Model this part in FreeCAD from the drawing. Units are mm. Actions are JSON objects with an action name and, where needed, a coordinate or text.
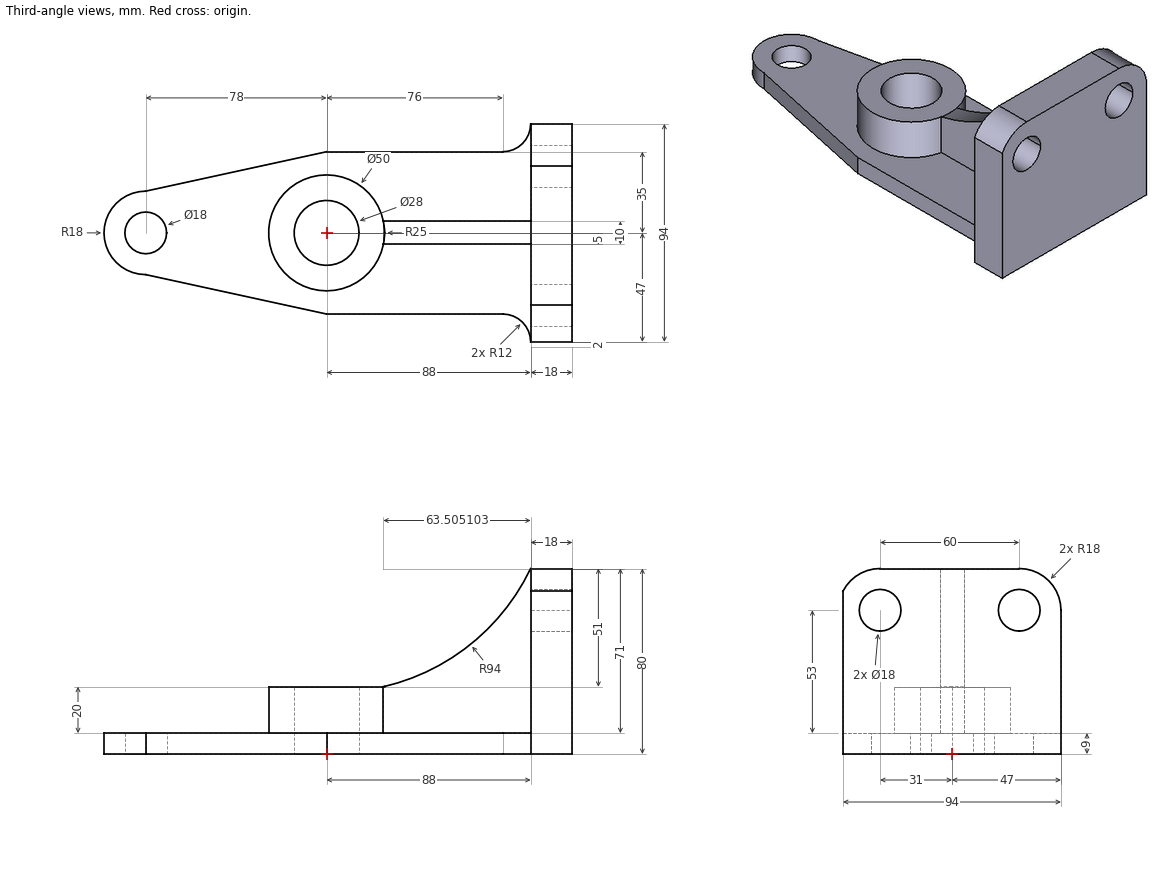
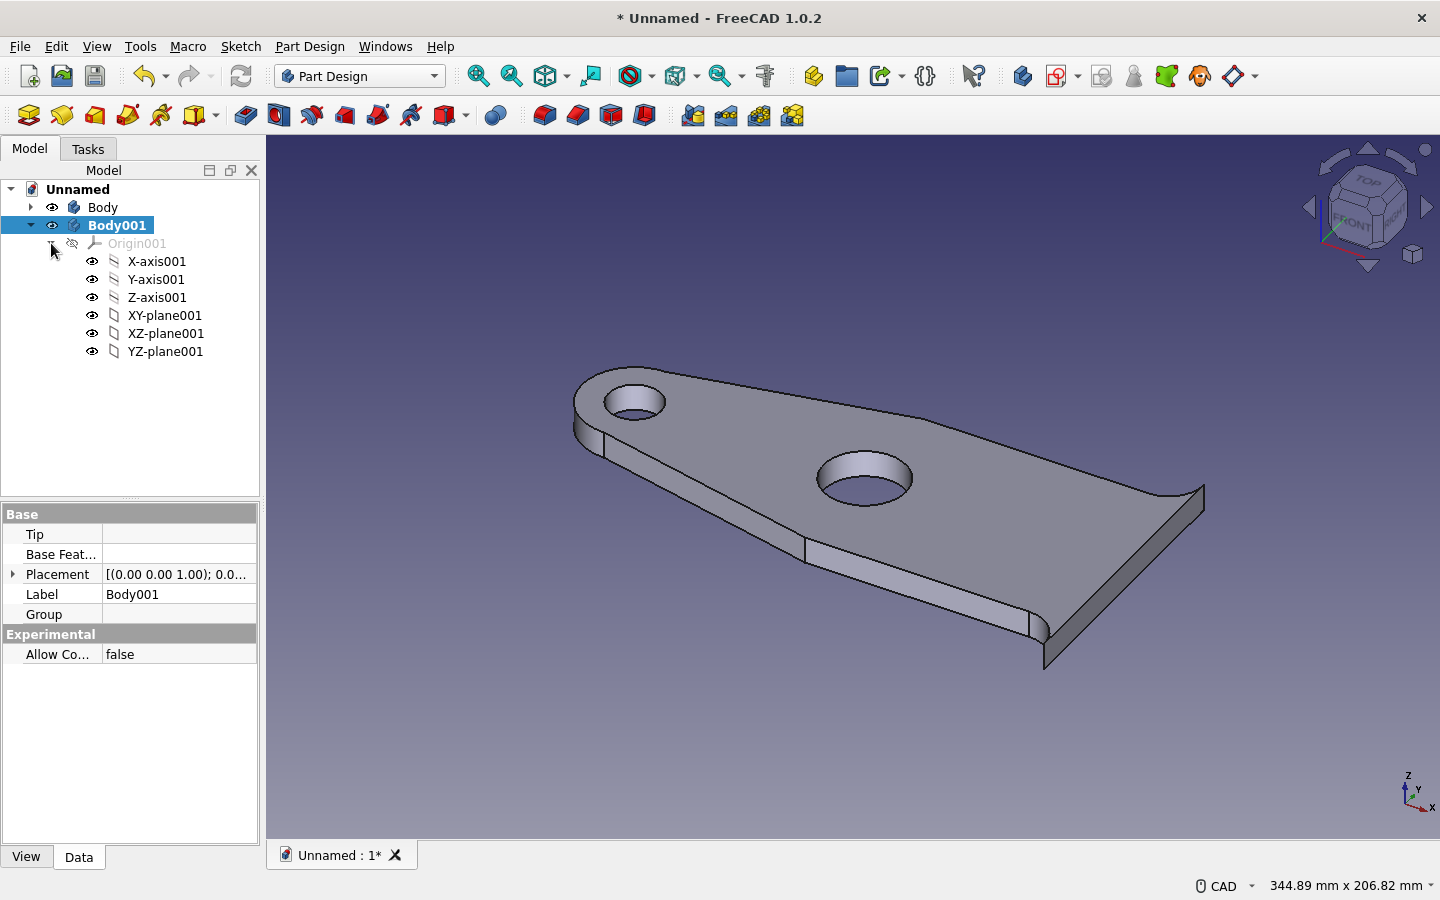
{"action": "left_click", "coordinate": [137, 351]}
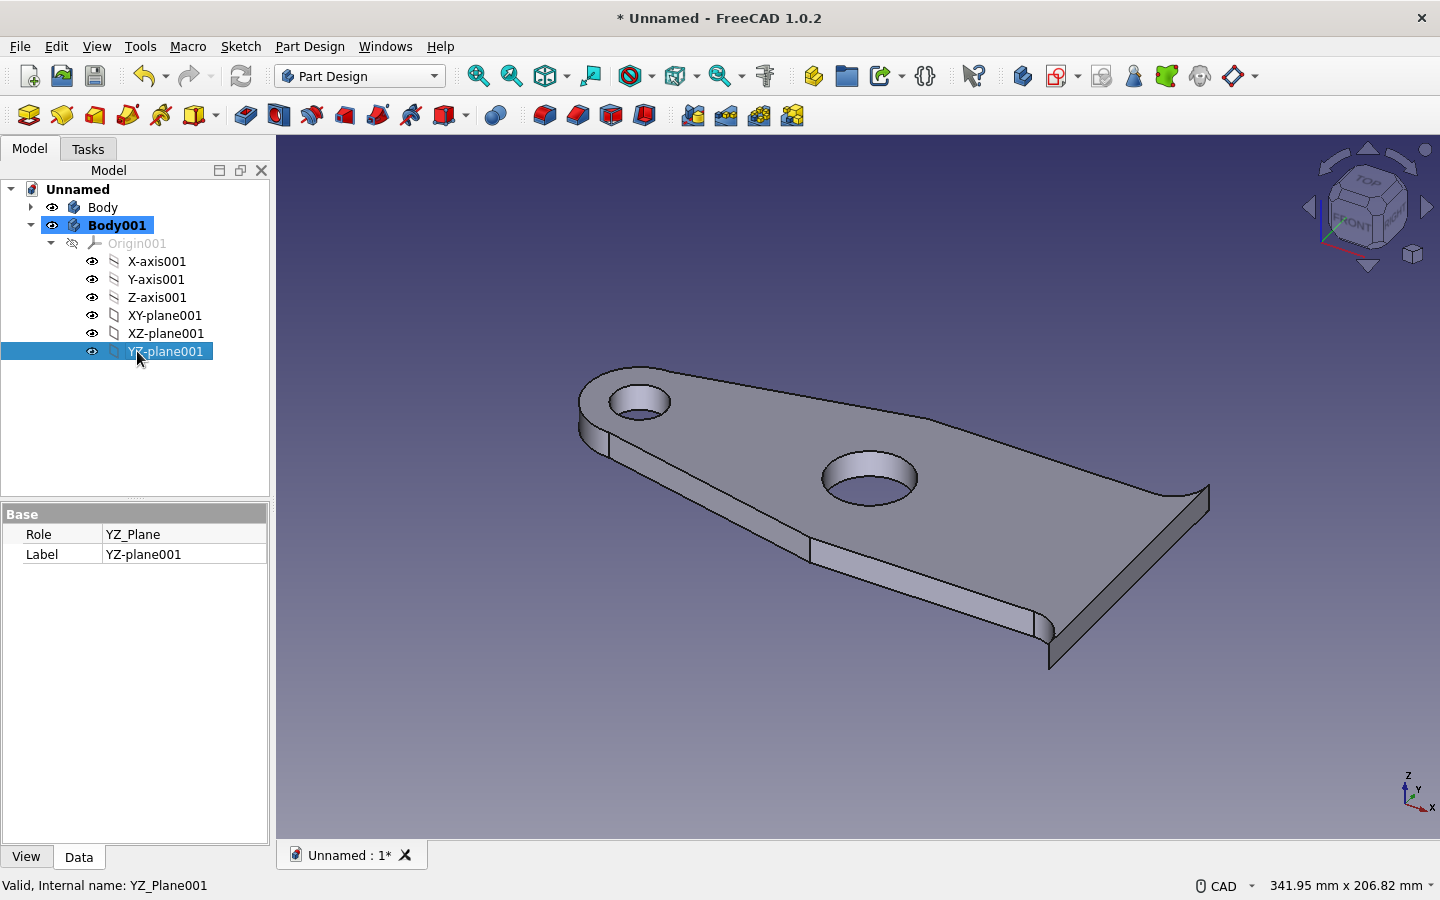
{"action": "left_click", "coordinate": [1232, 76]}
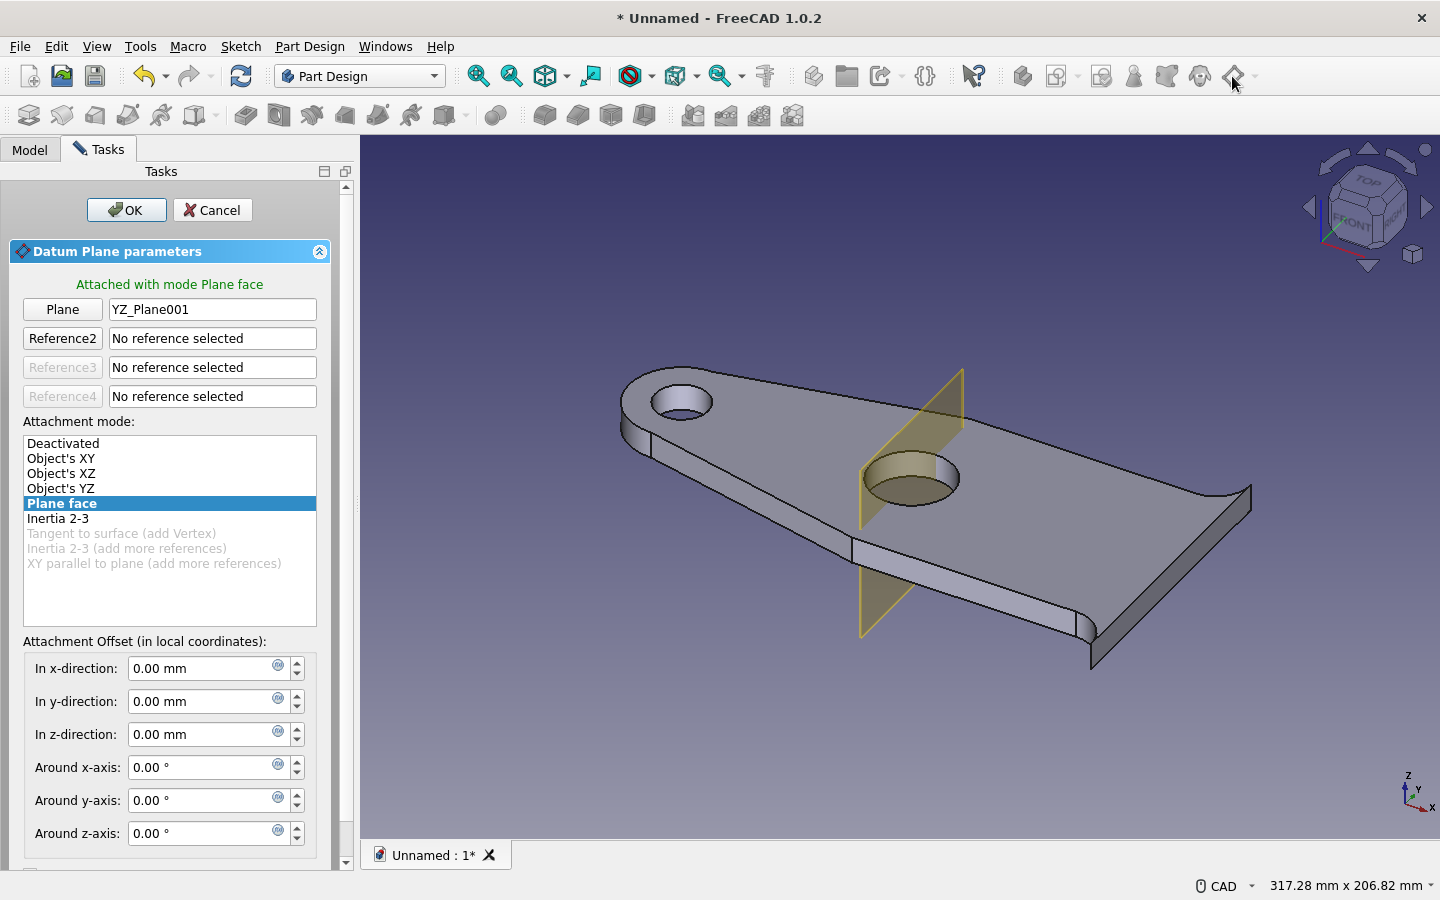
{"action": "triple_click", "coordinate": [210, 734]}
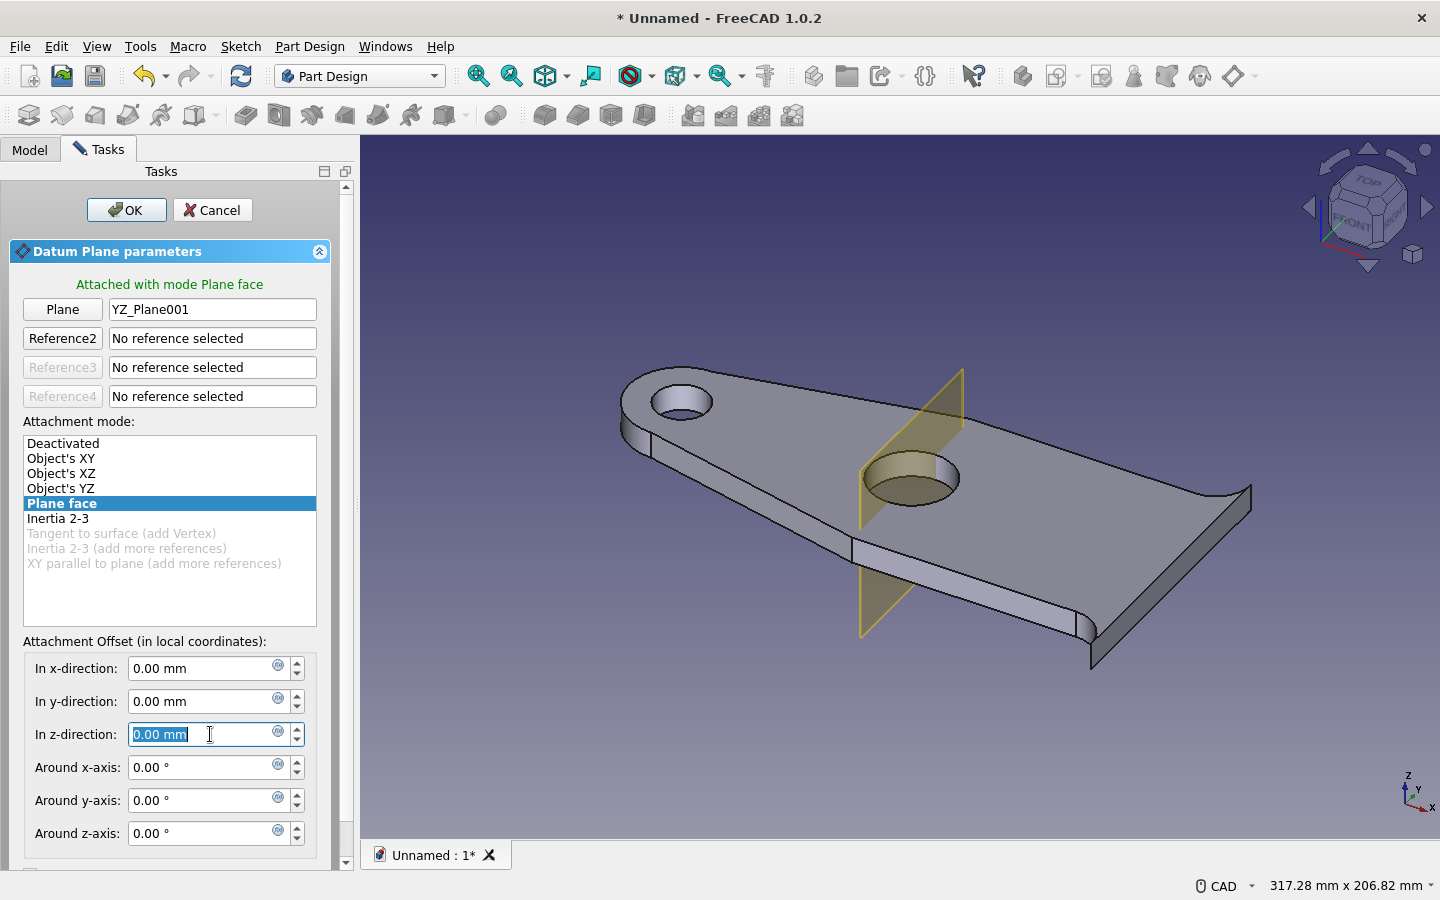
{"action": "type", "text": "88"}
{"action": "key", "text": "Tab"}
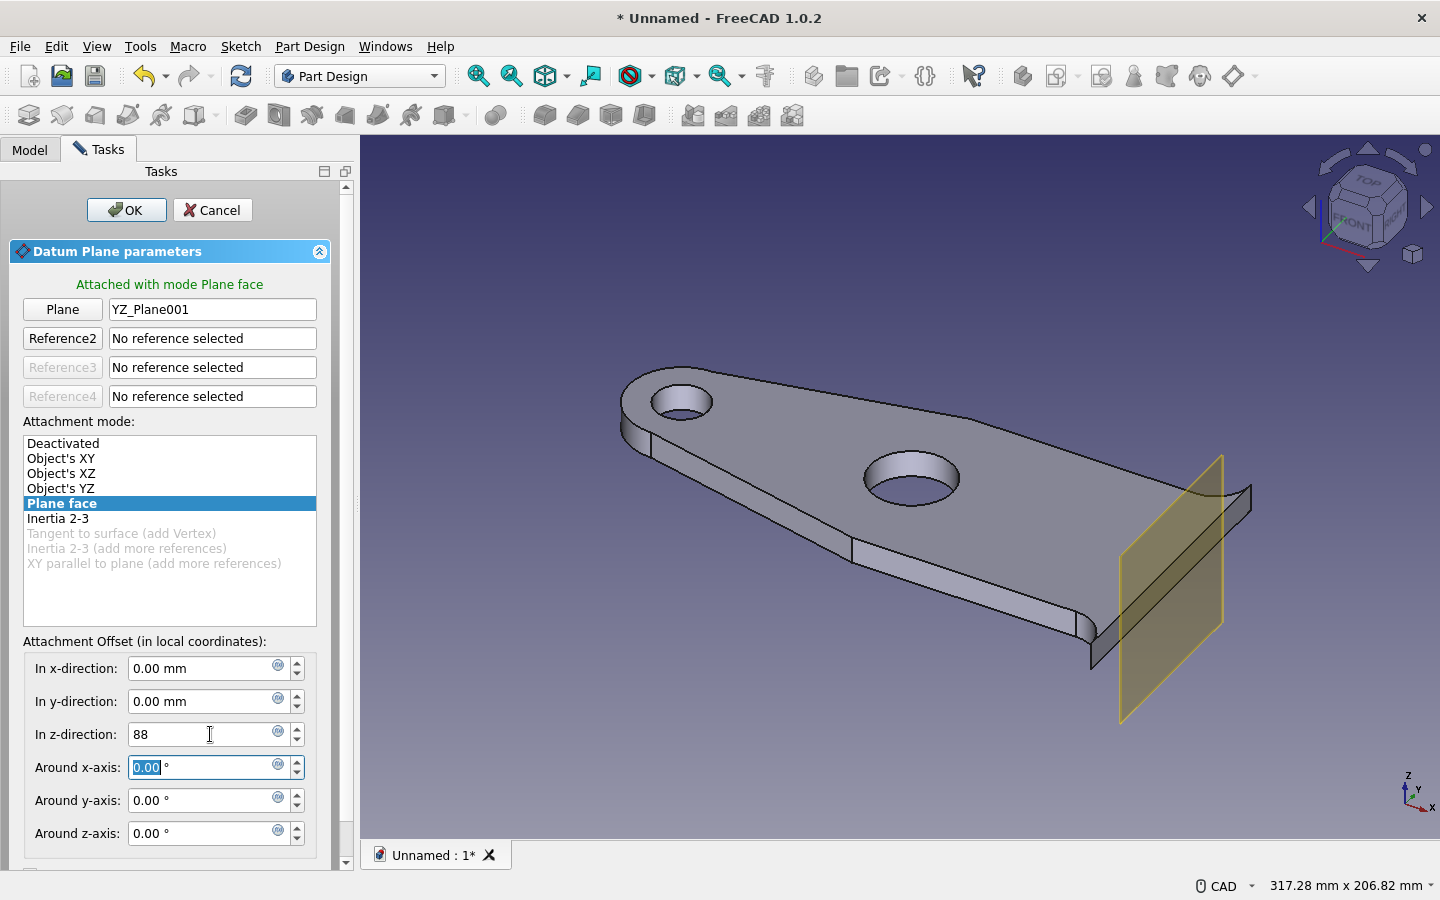
{"action": "left_click", "coordinate": [127, 210]}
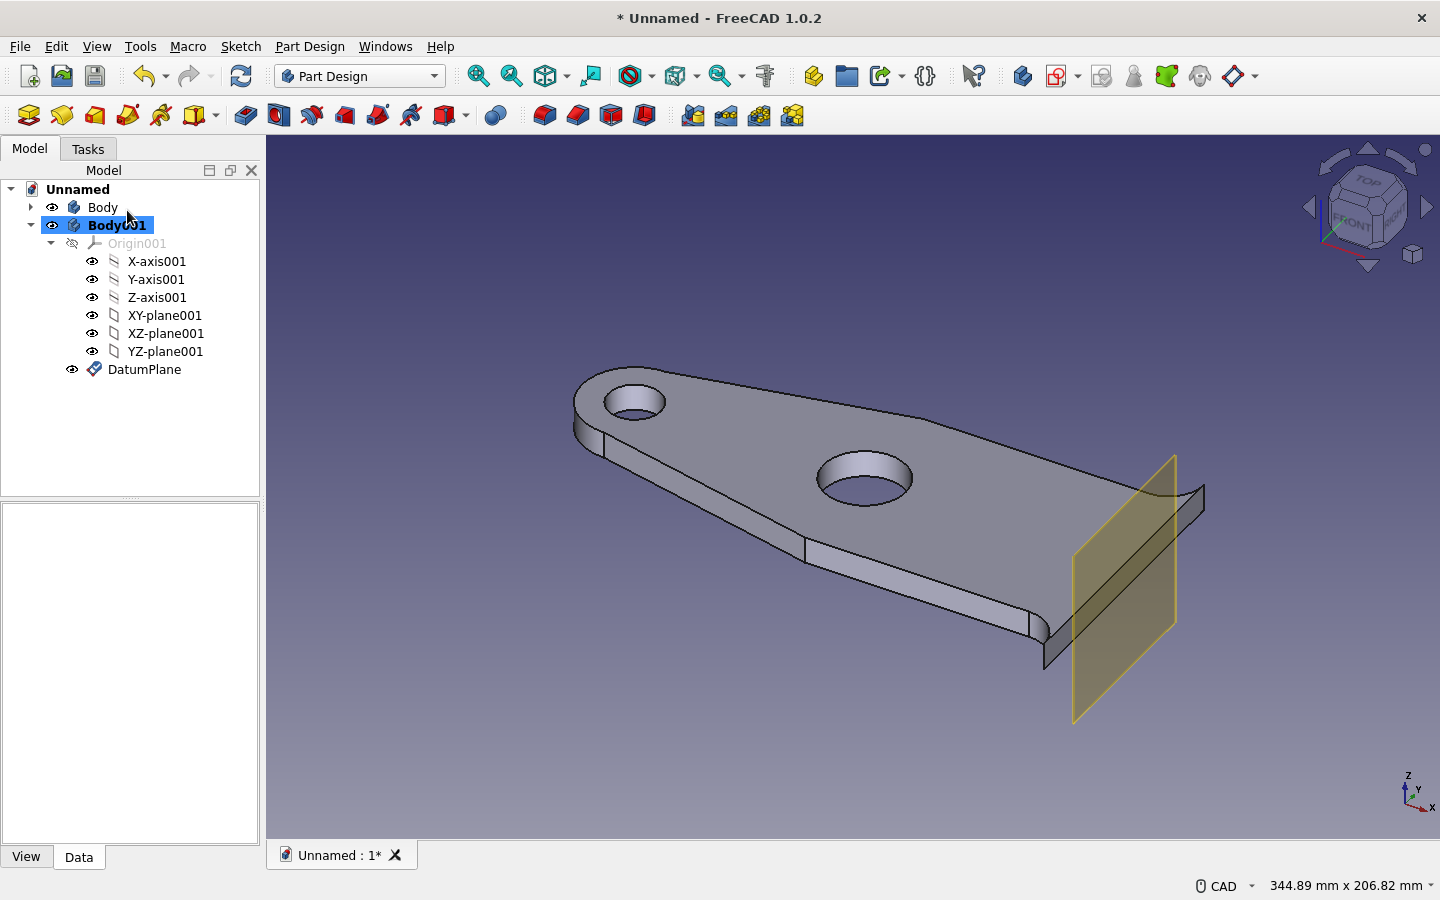
{"action": "left_click", "coordinate": [117, 369]}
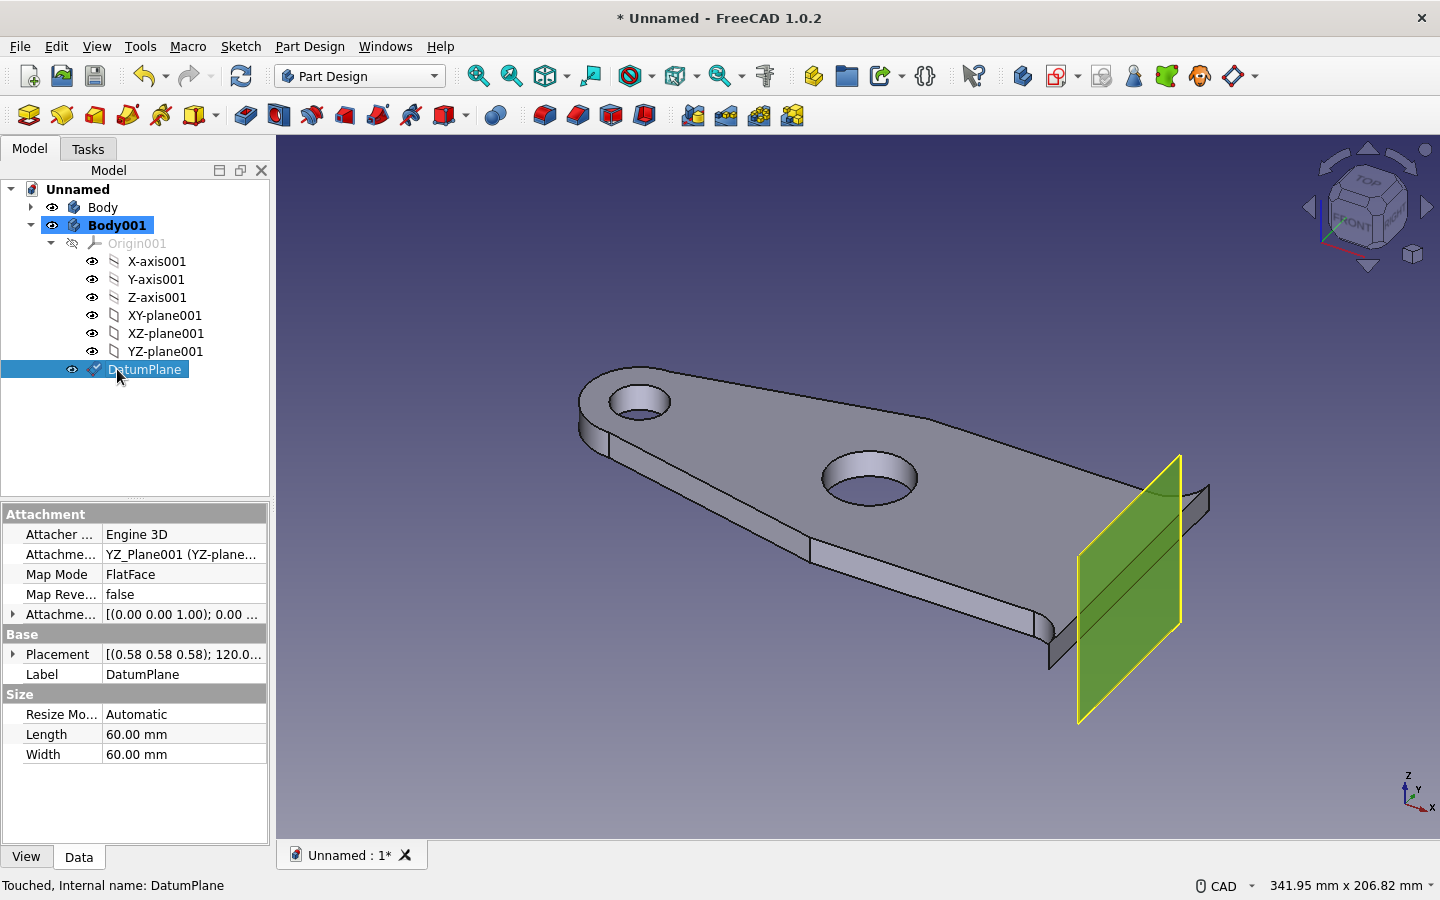
{"action": "left_click", "coordinate": [1056, 76]}